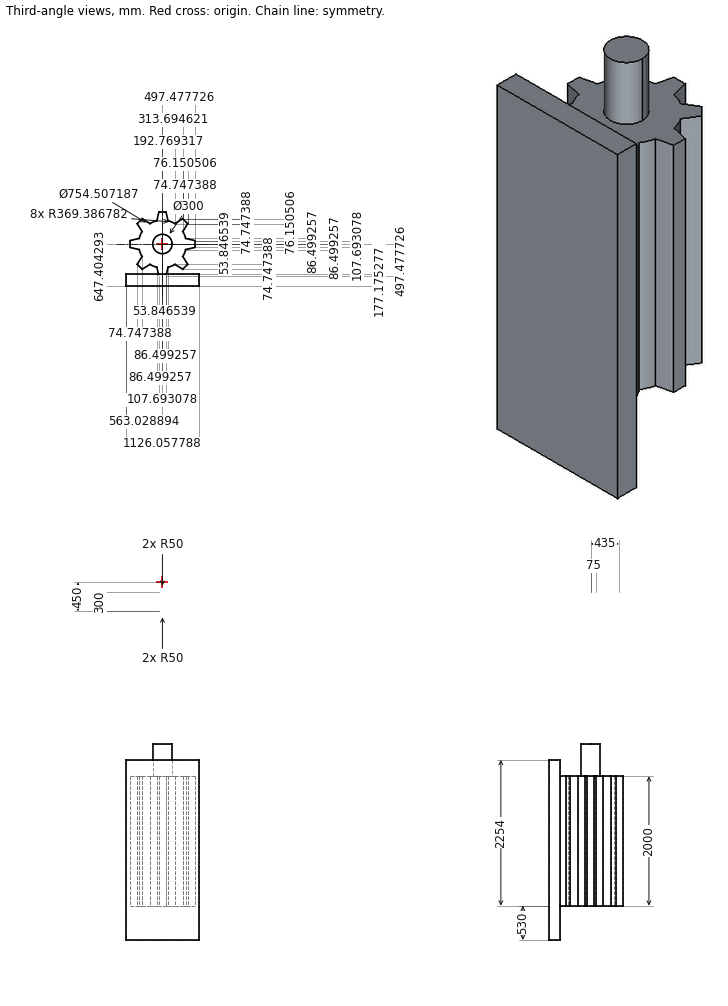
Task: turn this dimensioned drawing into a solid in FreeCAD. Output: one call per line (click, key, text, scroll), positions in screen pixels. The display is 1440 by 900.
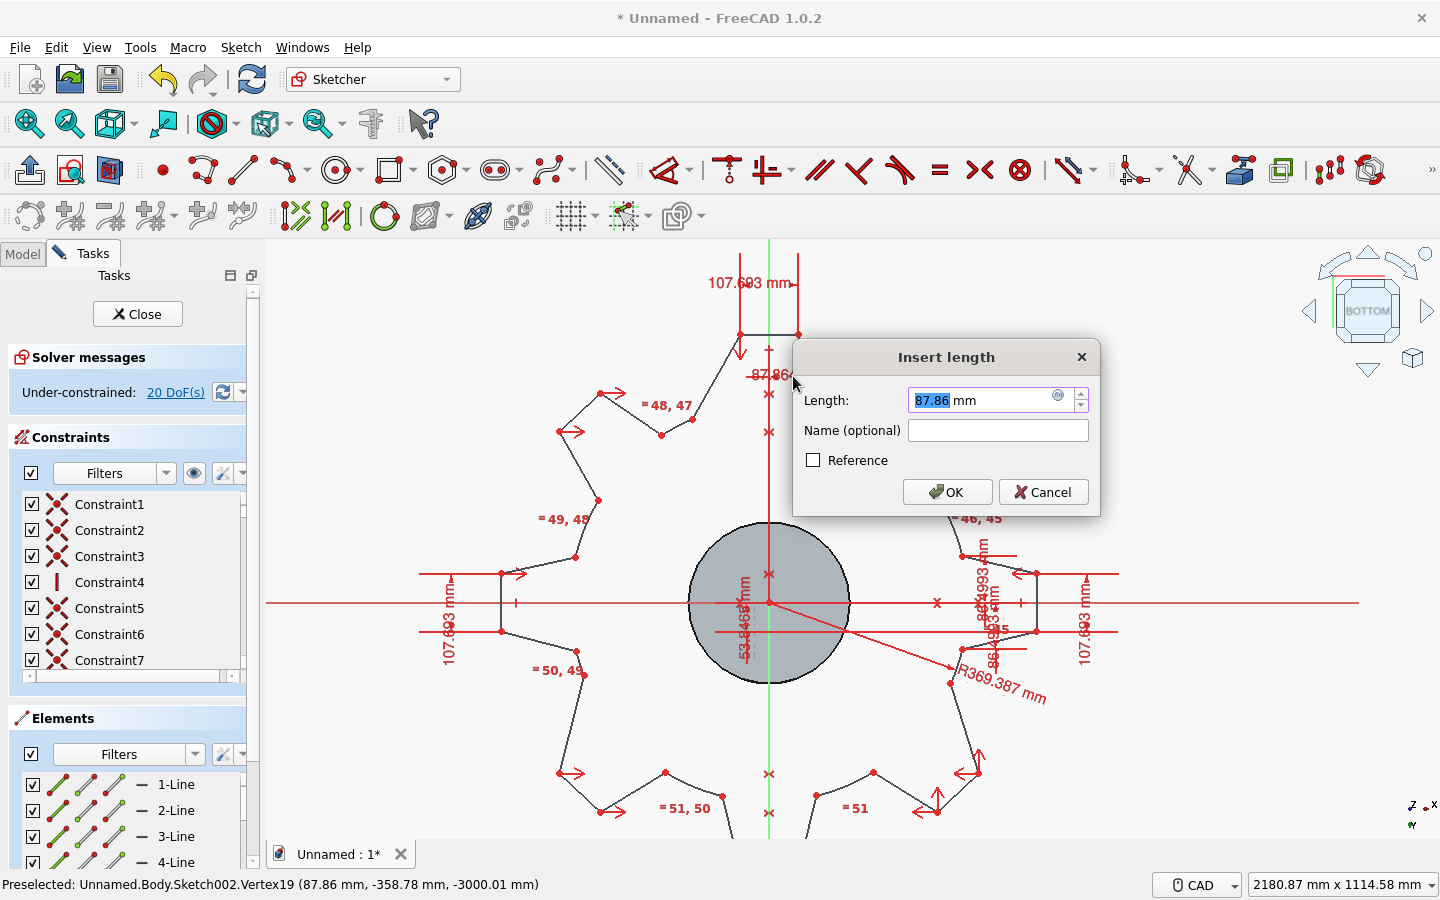
text(86.499257)
key(Return)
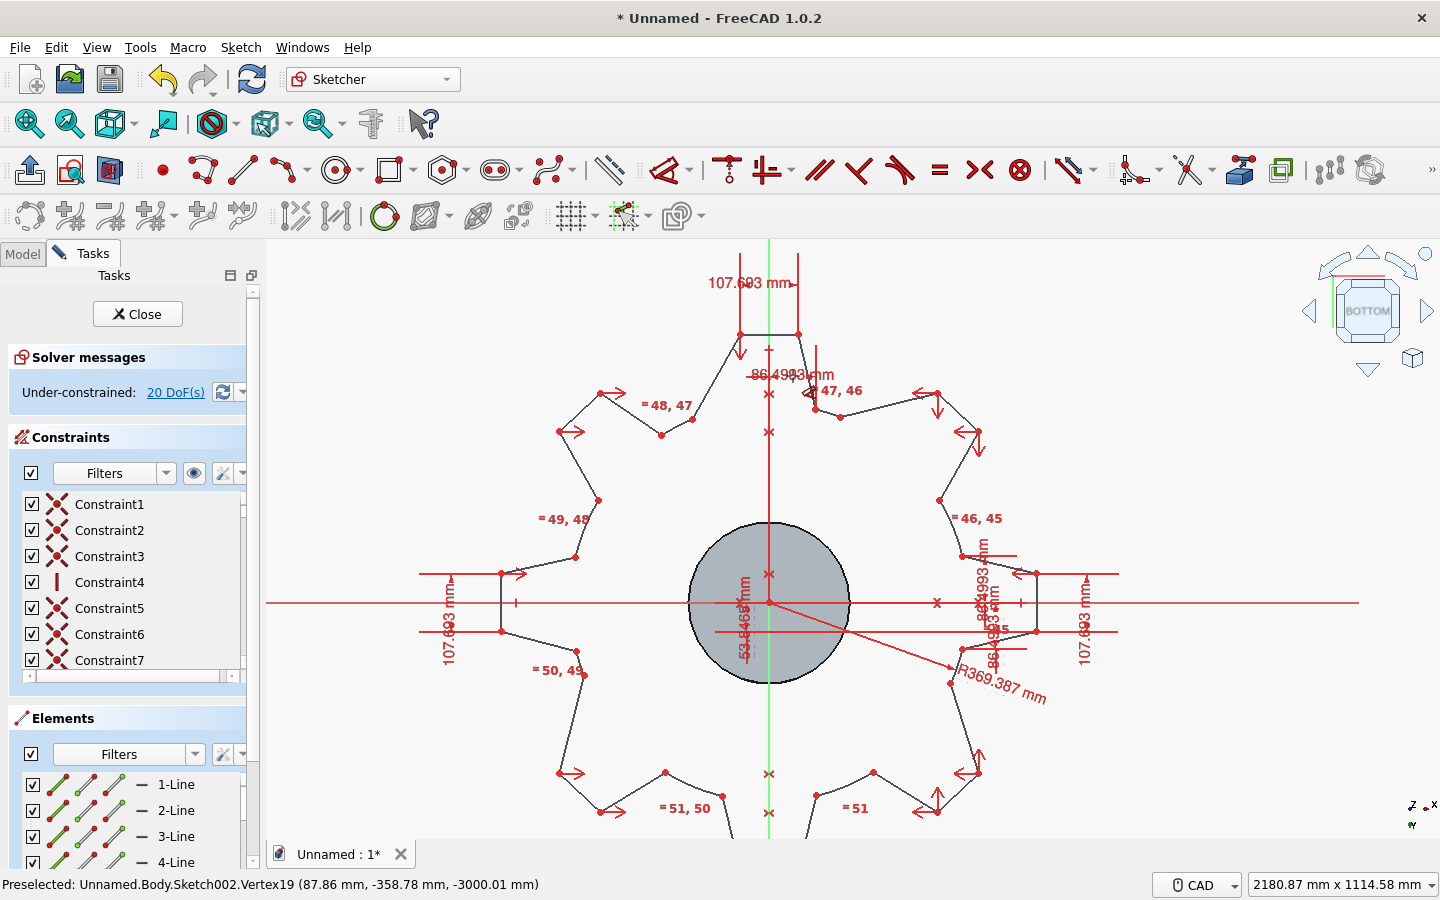
scroll(798, 335, up, 2)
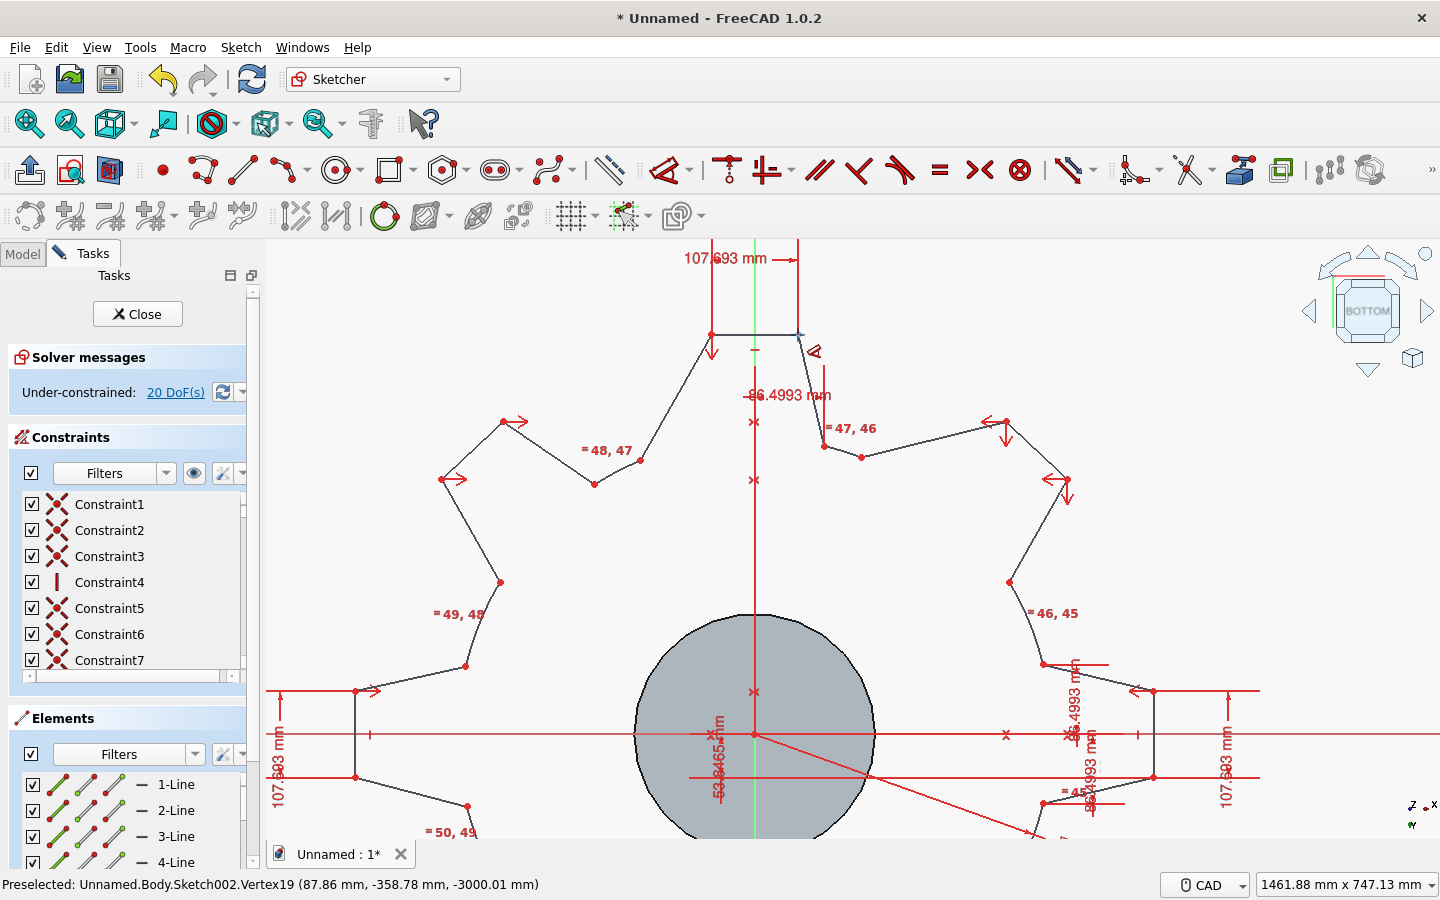
click(798, 335)
click(776, 301)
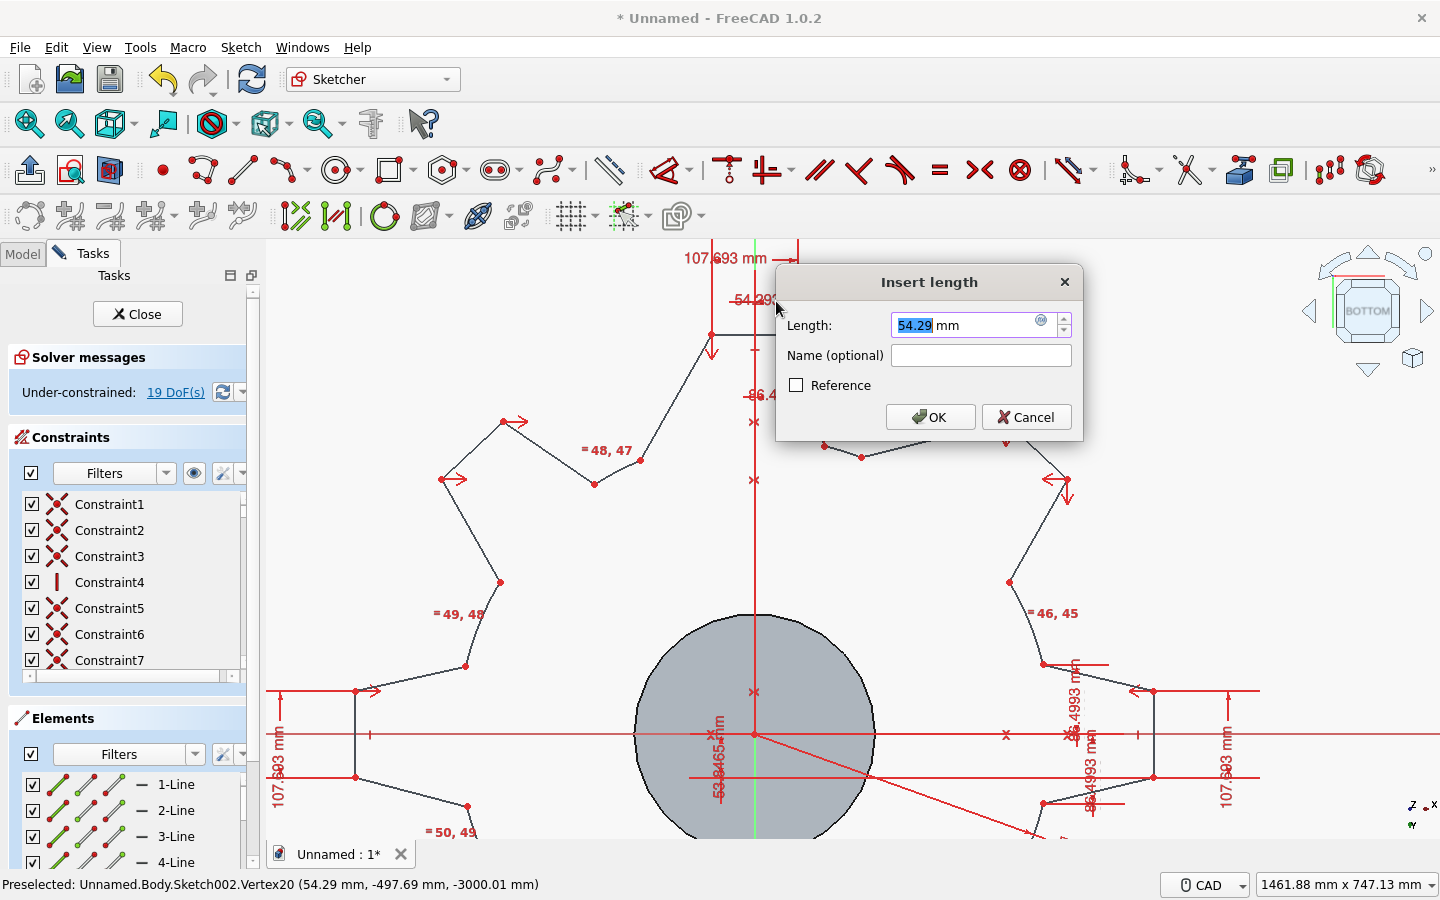
text(53.846539)
key(Return)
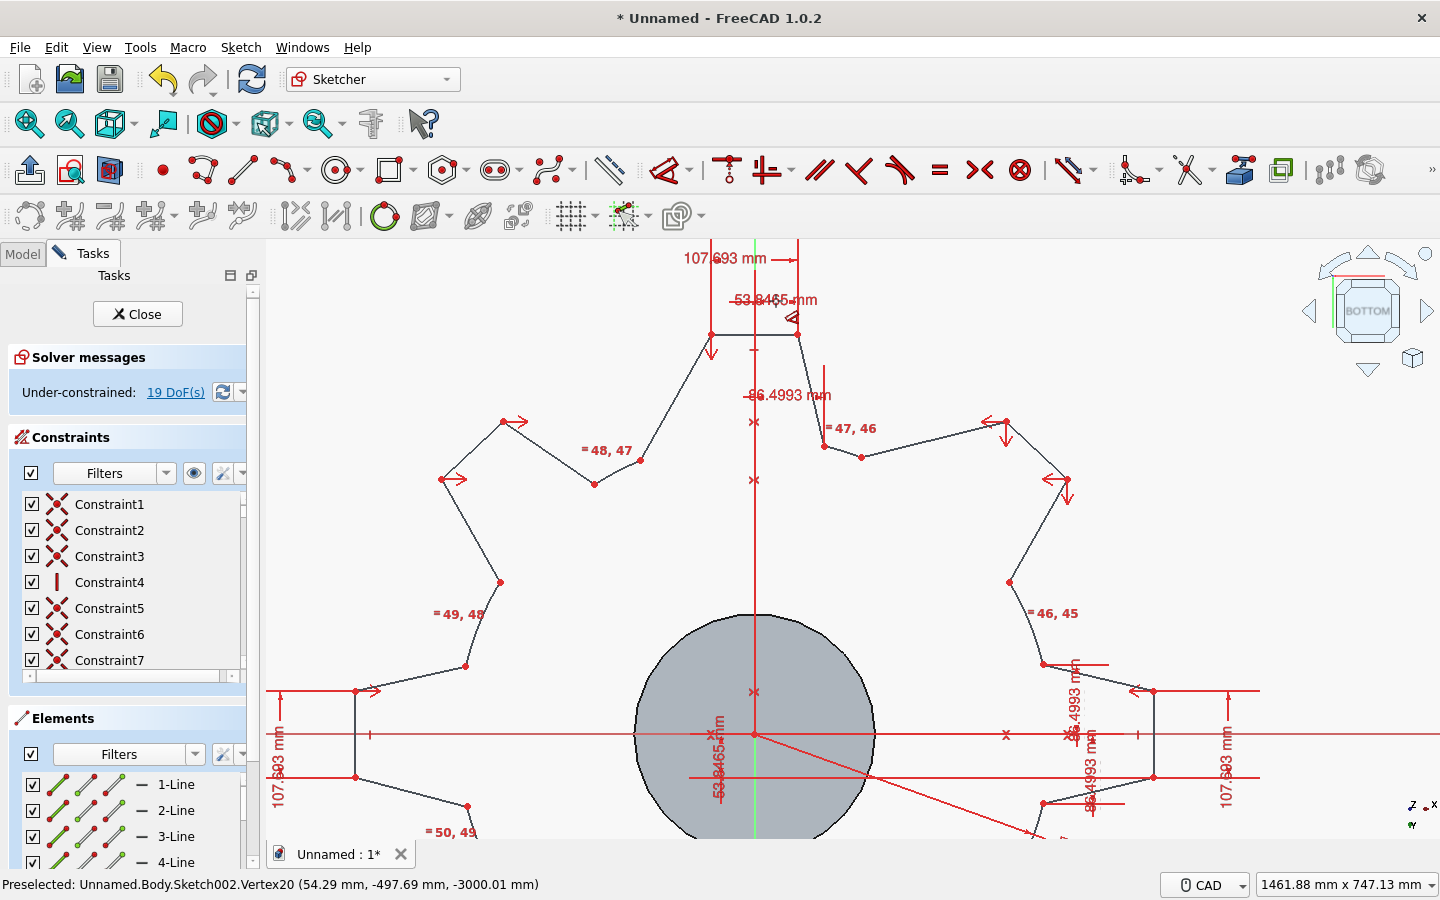
click(640, 461)
click(697, 427)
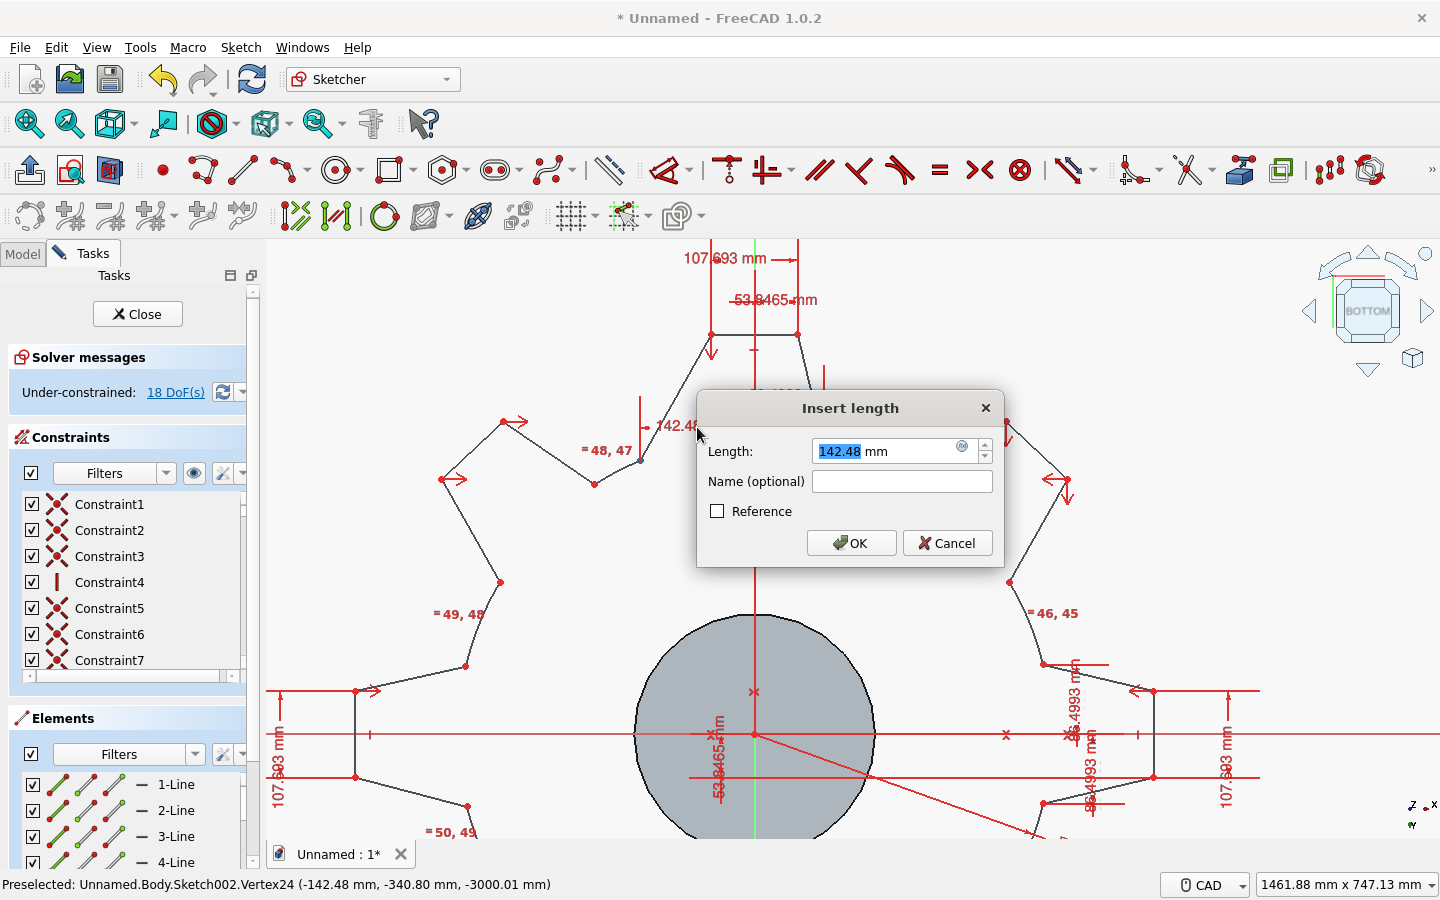
text(86.499257)
key(Return)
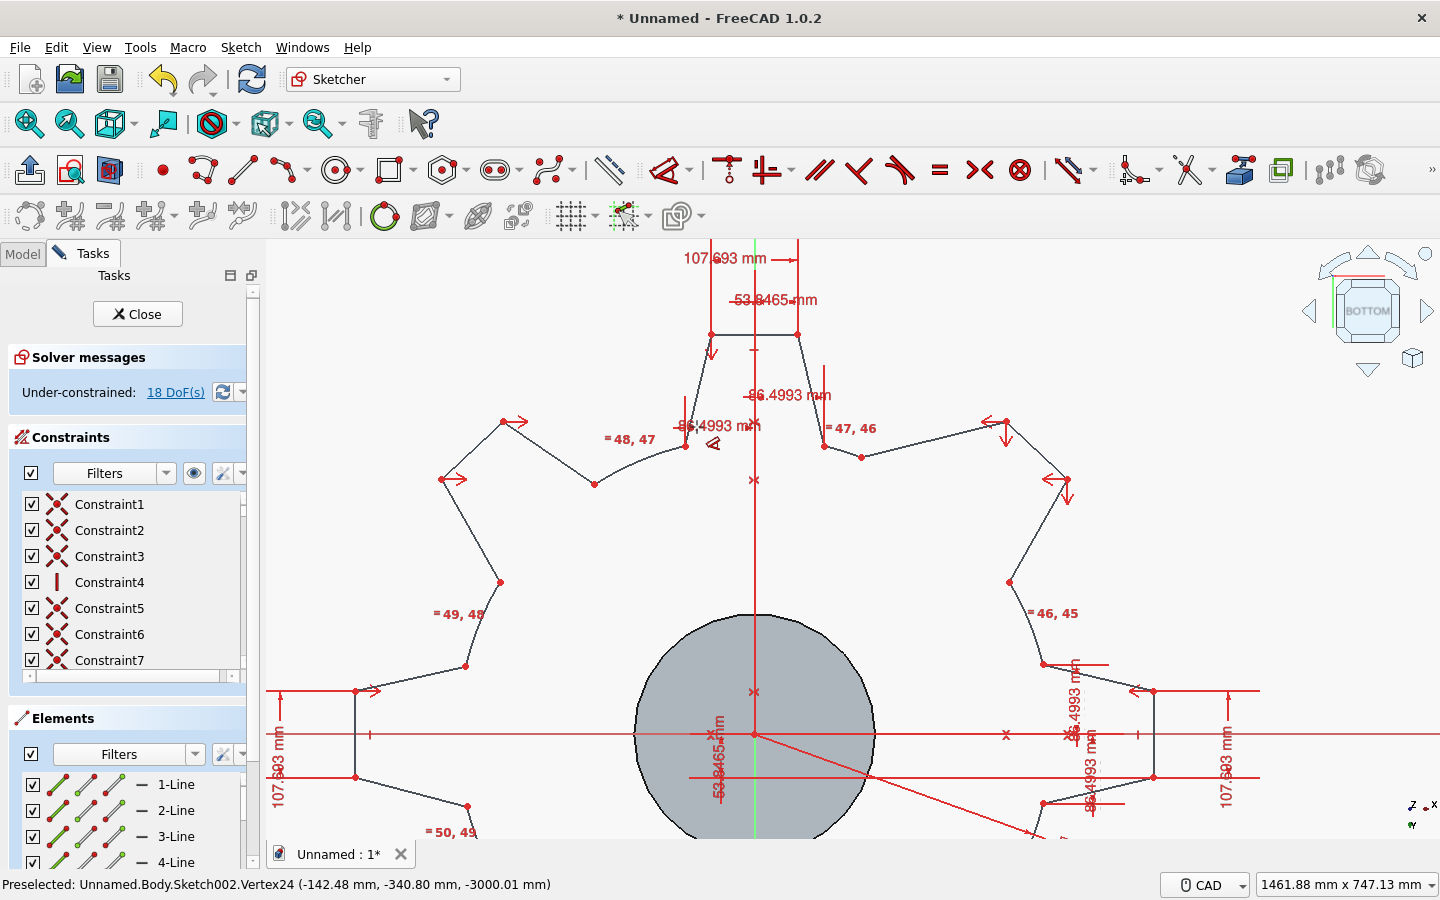
click(466, 667)
click(432, 701)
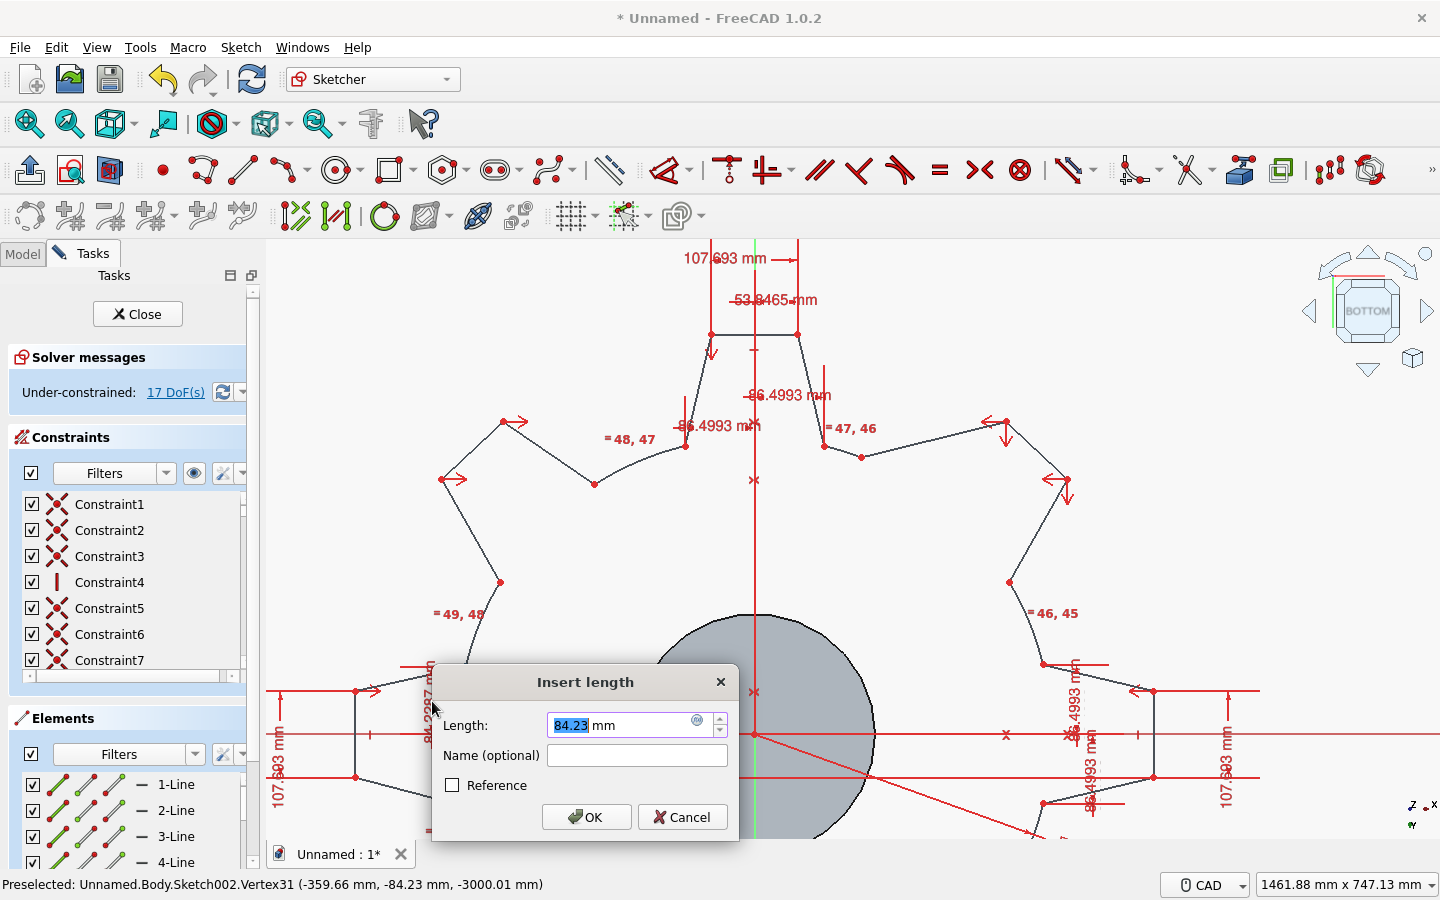
text(86.499257)
key(Return)